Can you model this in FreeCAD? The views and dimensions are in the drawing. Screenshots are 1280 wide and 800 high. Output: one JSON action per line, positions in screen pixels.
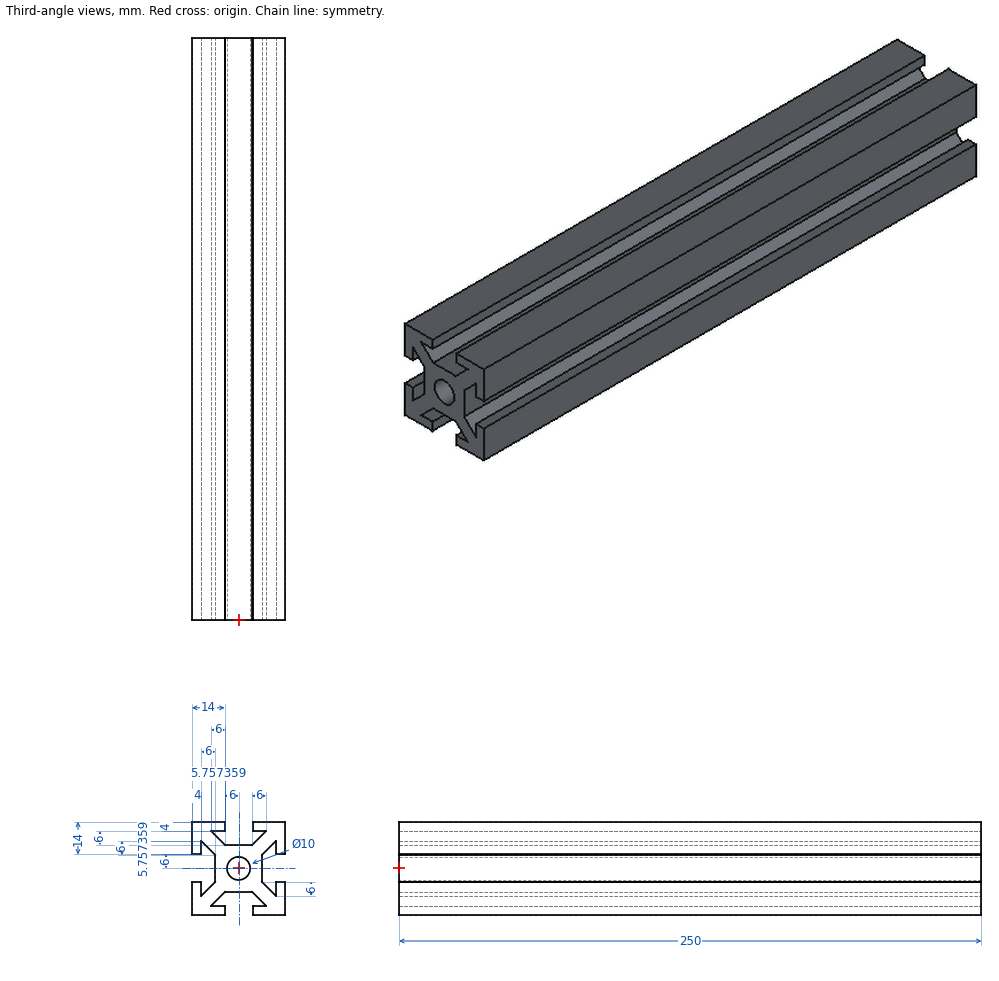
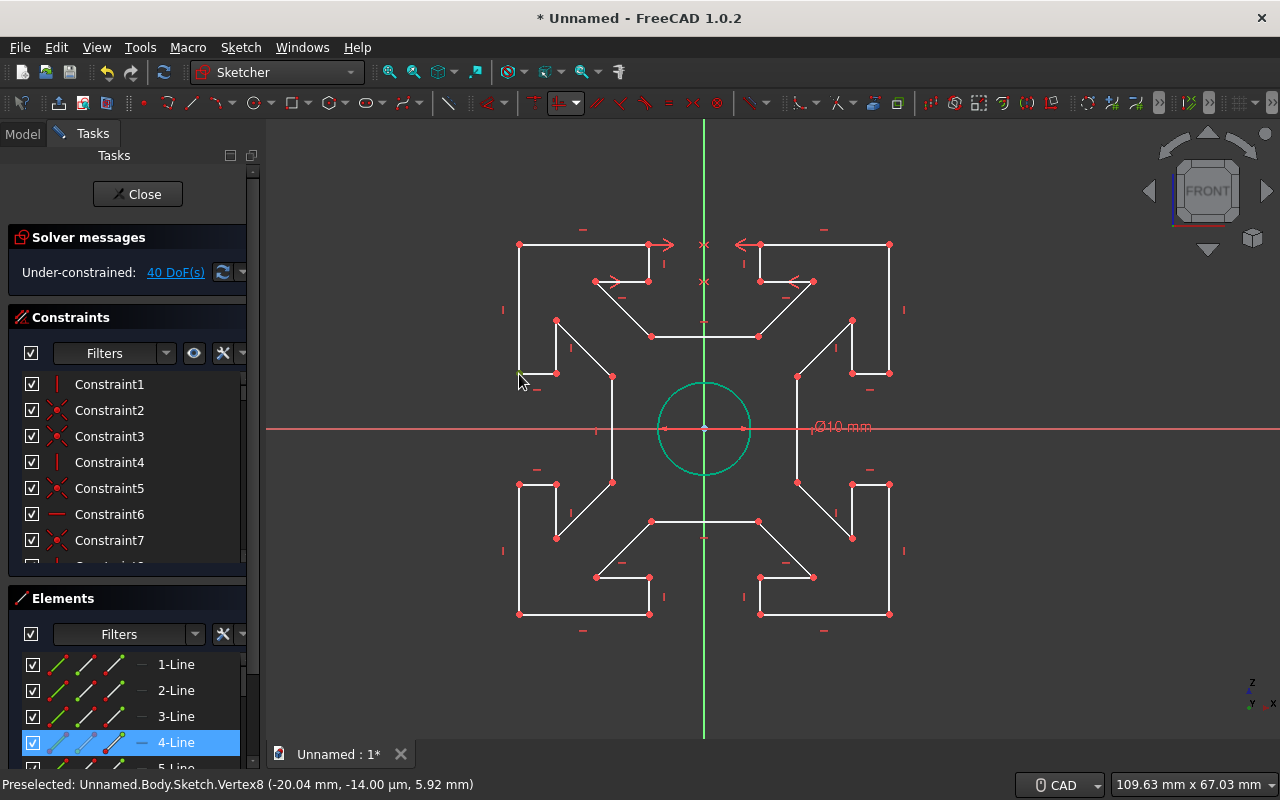
{"action": "left_click", "coordinate": [889, 374]}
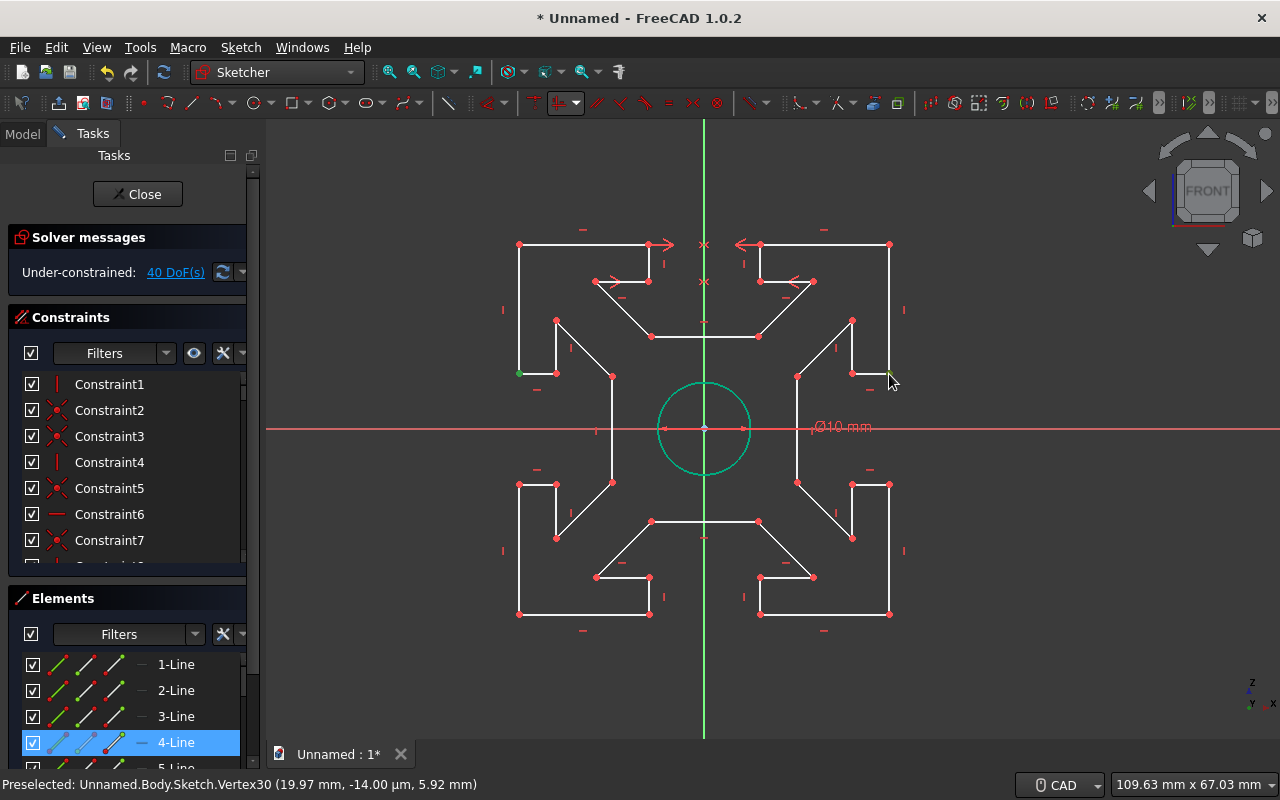
{"action": "left_click", "coordinate": [704, 671]}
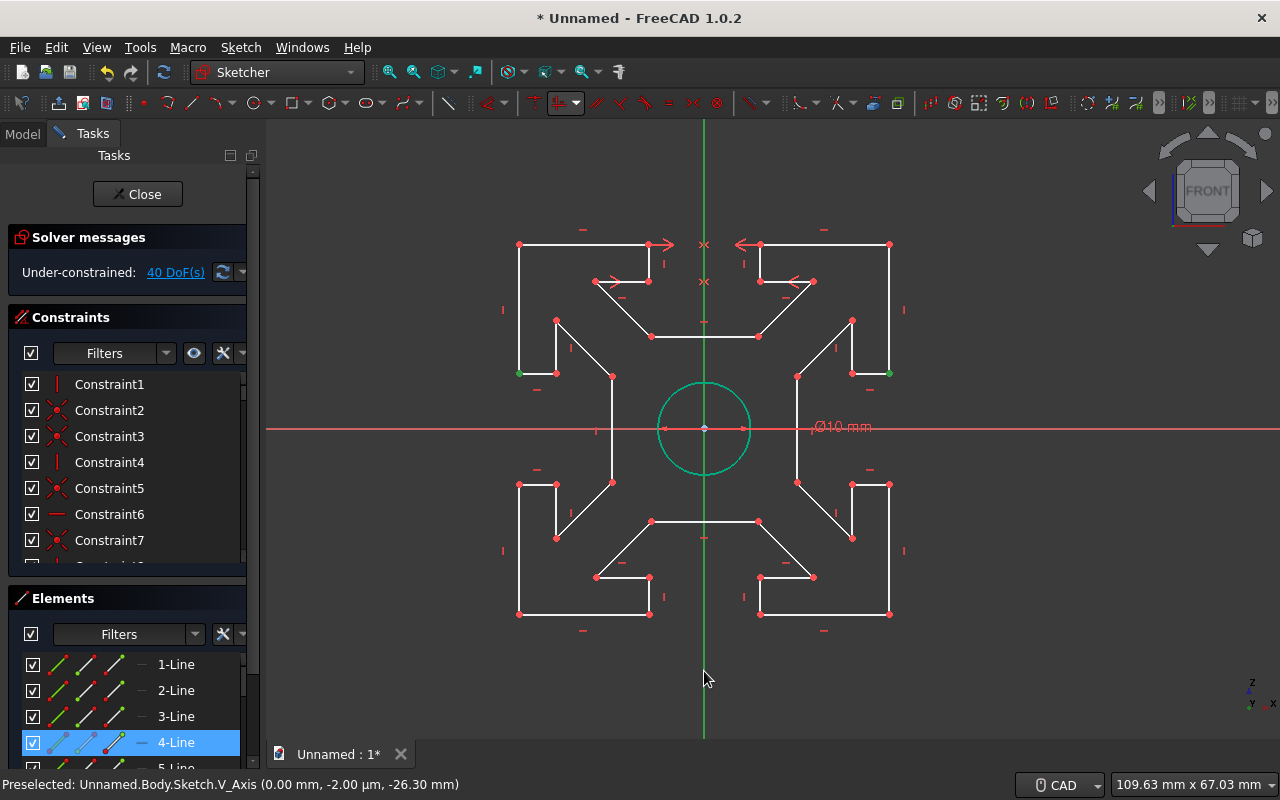
{"action": "left_click", "coordinate": [694, 104]}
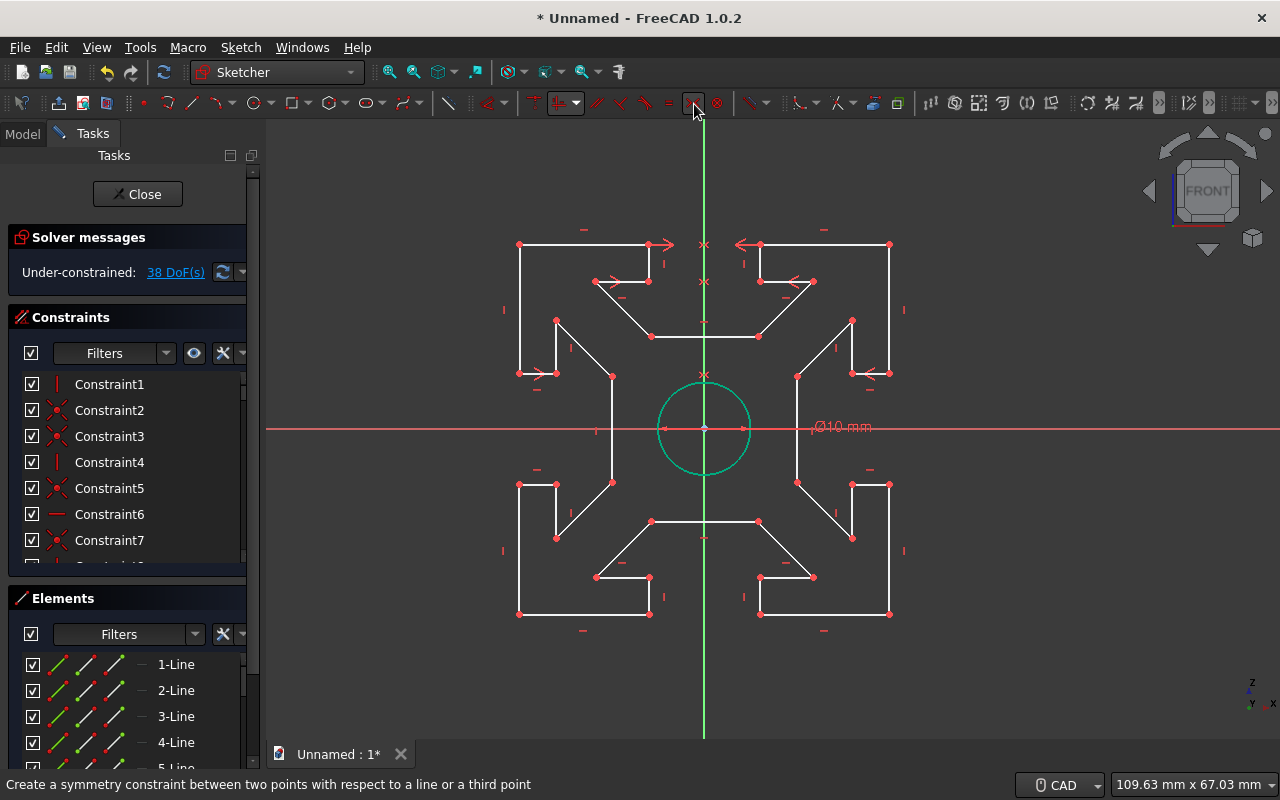
{"action": "left_click", "coordinate": [556, 321]}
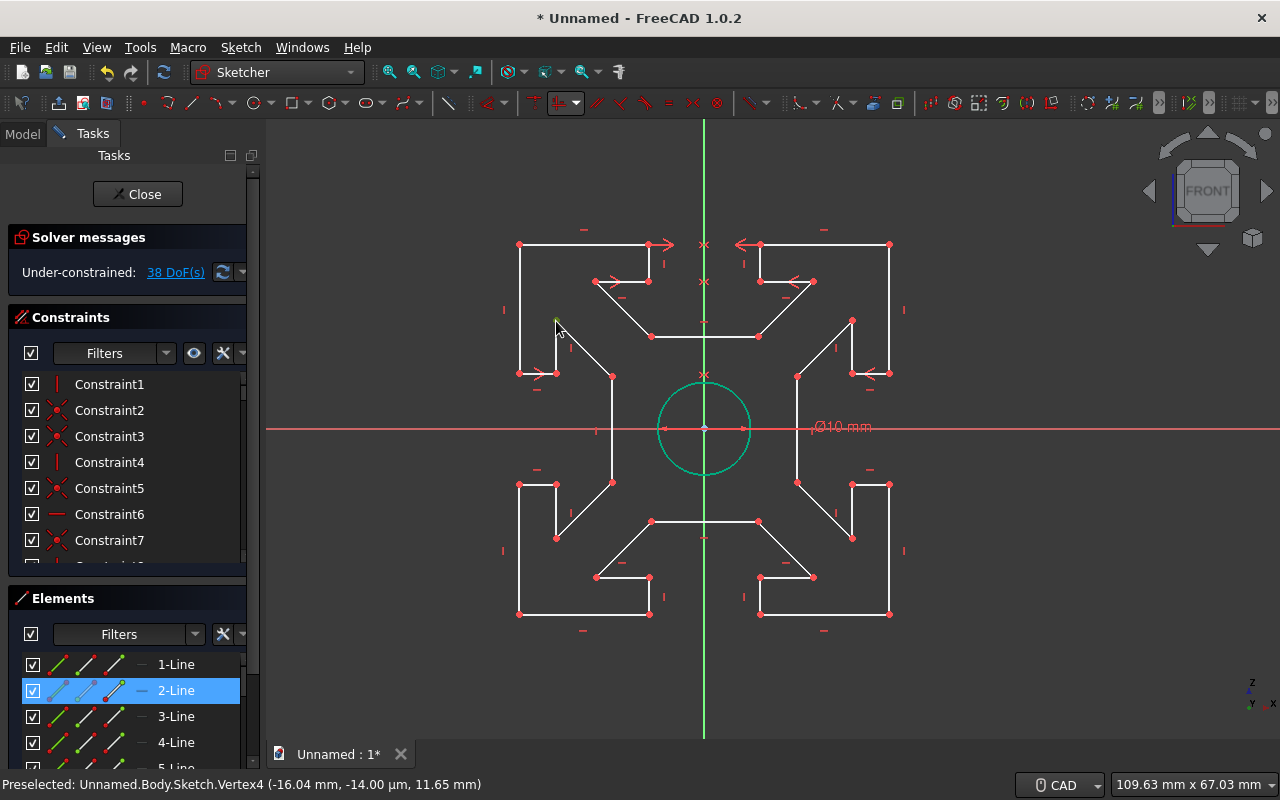
{"action": "left_click", "coordinate": [852, 321]}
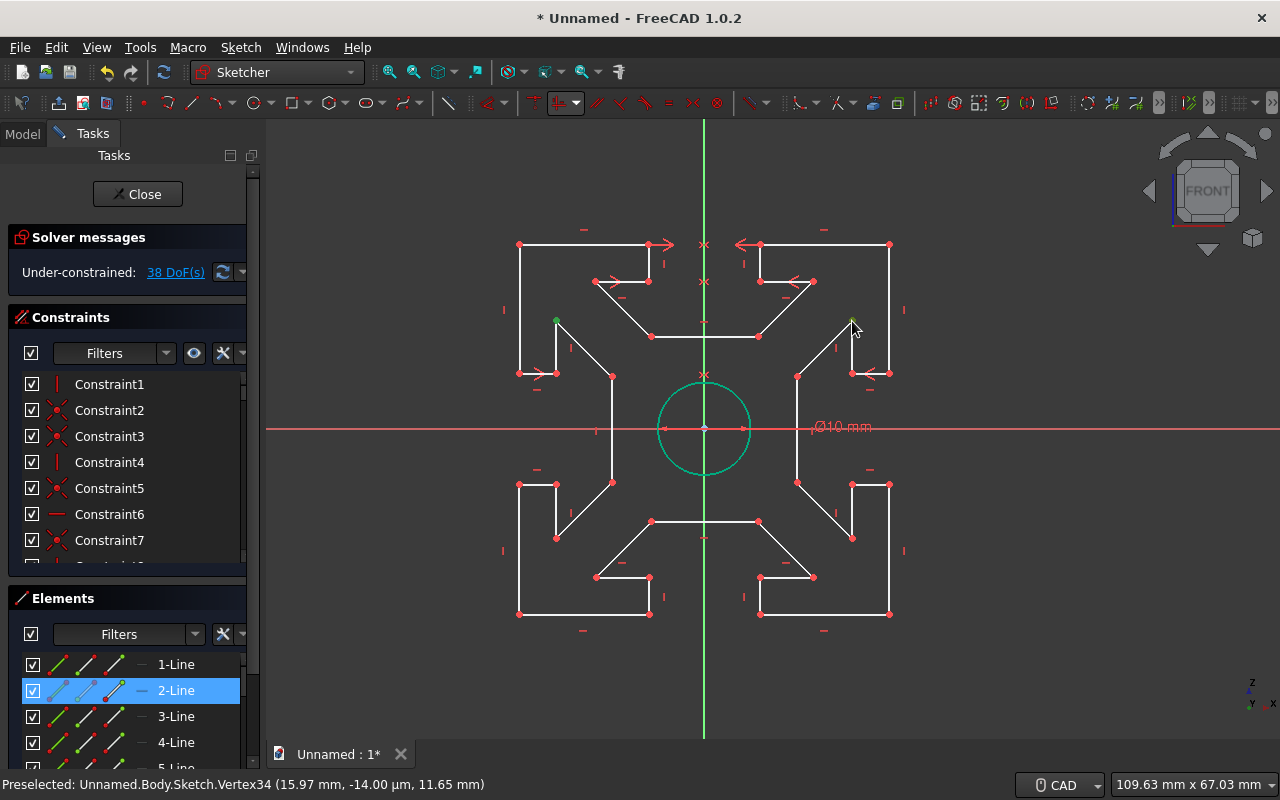
{"action": "left_click", "coordinate": [704, 671]}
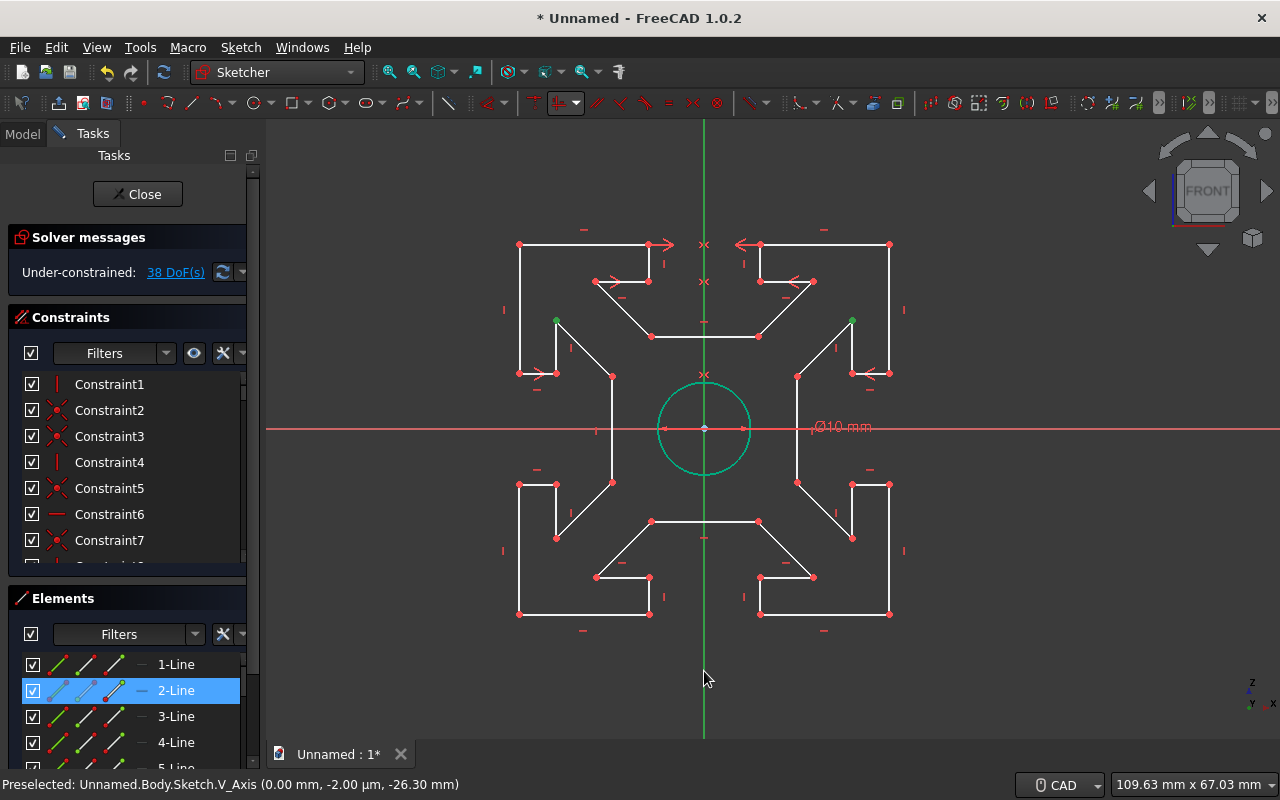
{"action": "left_click", "coordinate": [694, 104]}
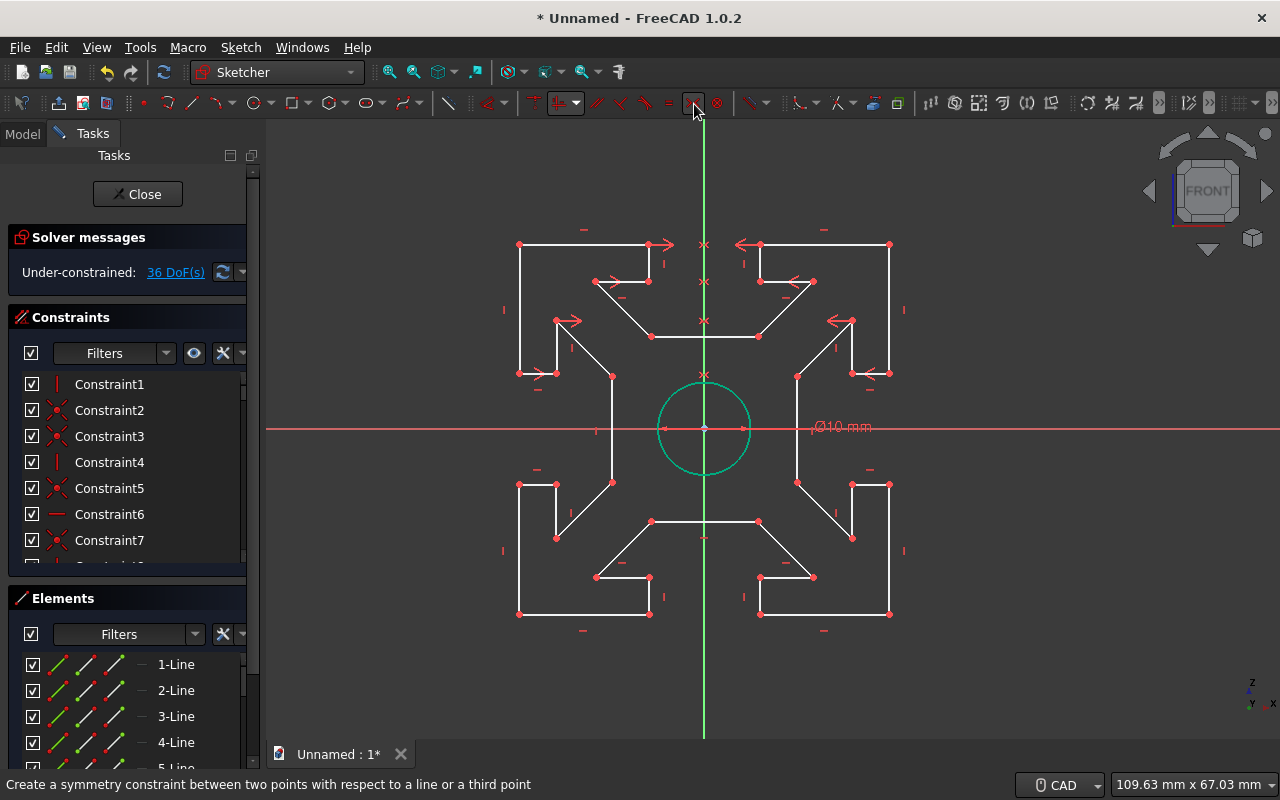
{"action": "left_click", "coordinate": [612, 377]}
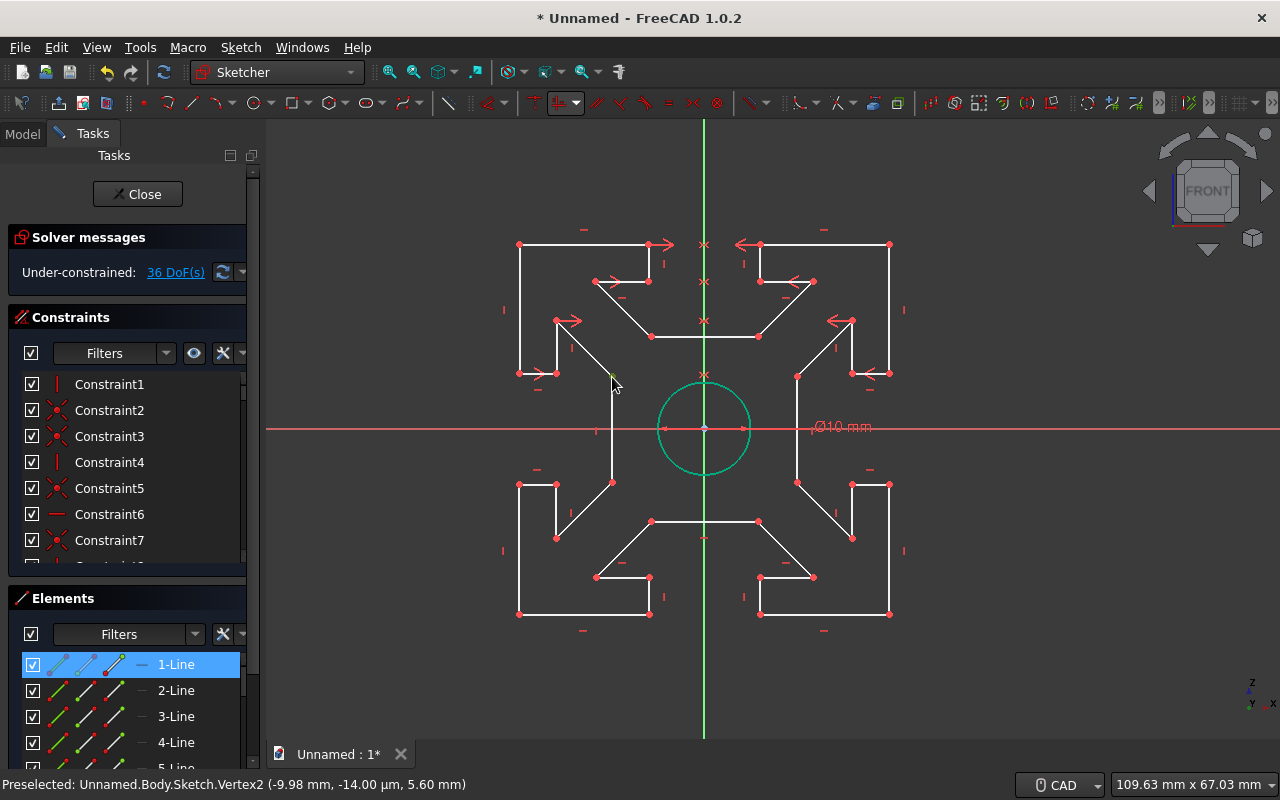
{"action": "left_click", "coordinate": [797, 377]}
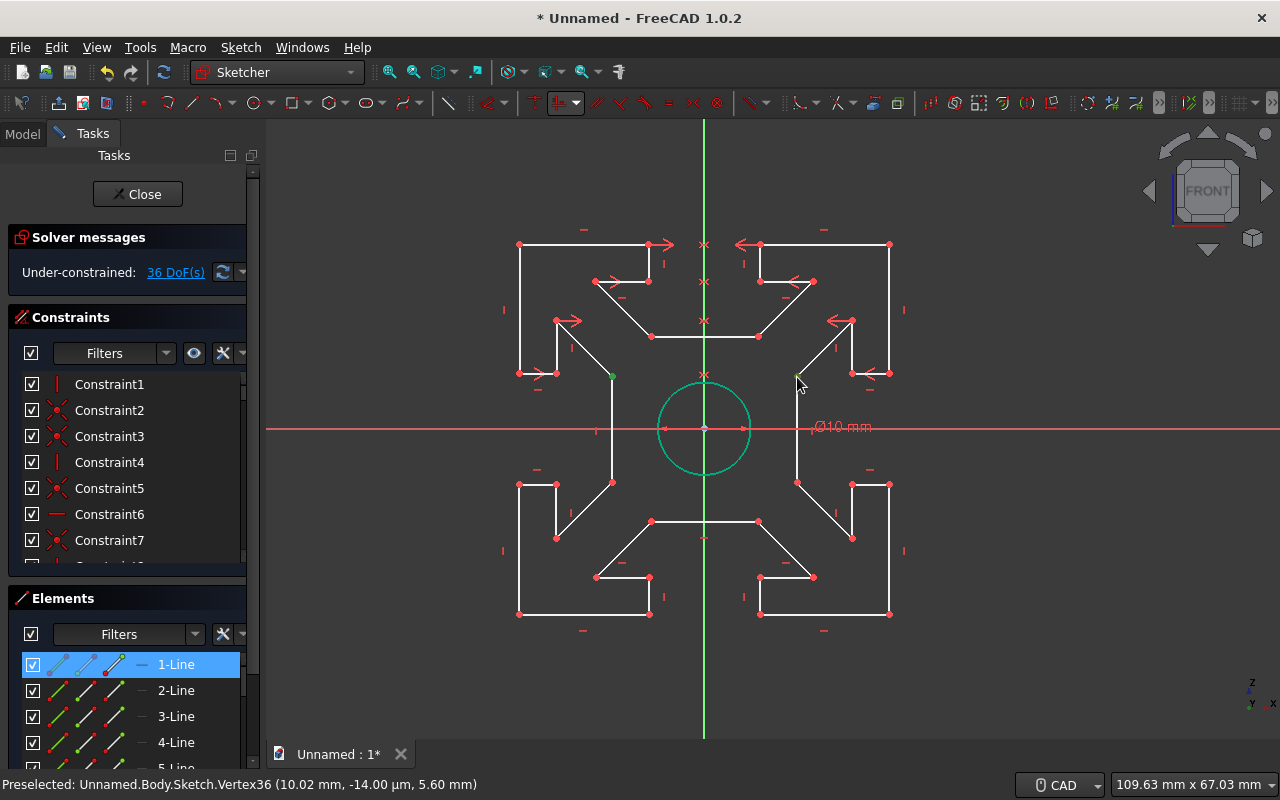
{"action": "left_click", "coordinate": [704, 671]}